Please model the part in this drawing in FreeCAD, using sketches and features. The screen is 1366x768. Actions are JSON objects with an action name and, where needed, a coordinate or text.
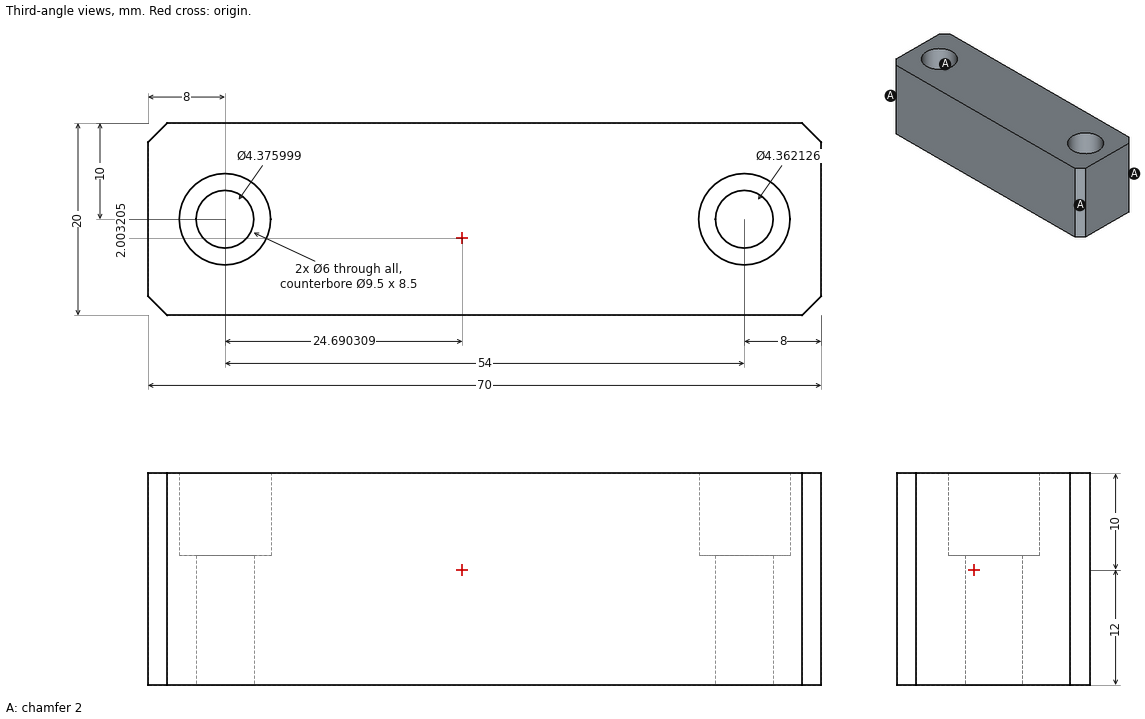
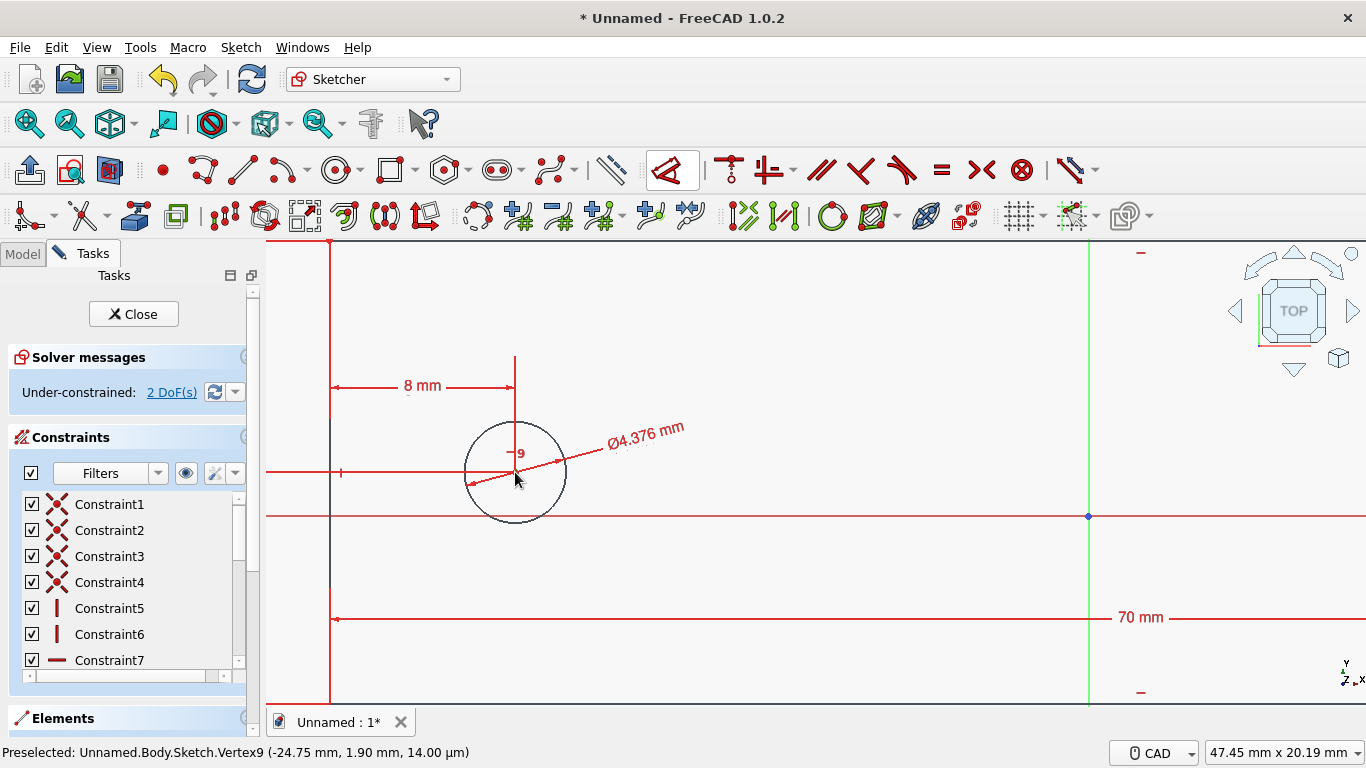
{"action": "key", "text": "i"}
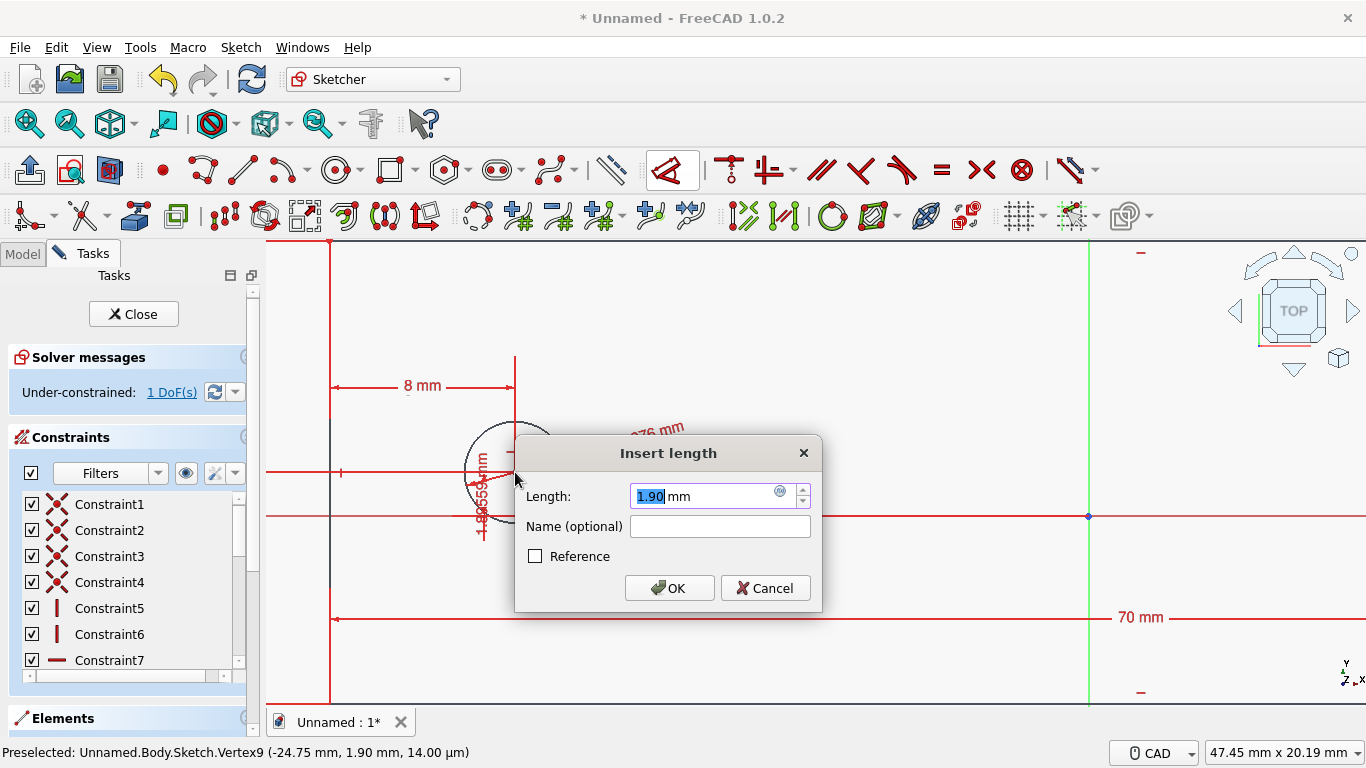
{"action": "type", "text": "2.003205"}
{"action": "key", "text": "Return"}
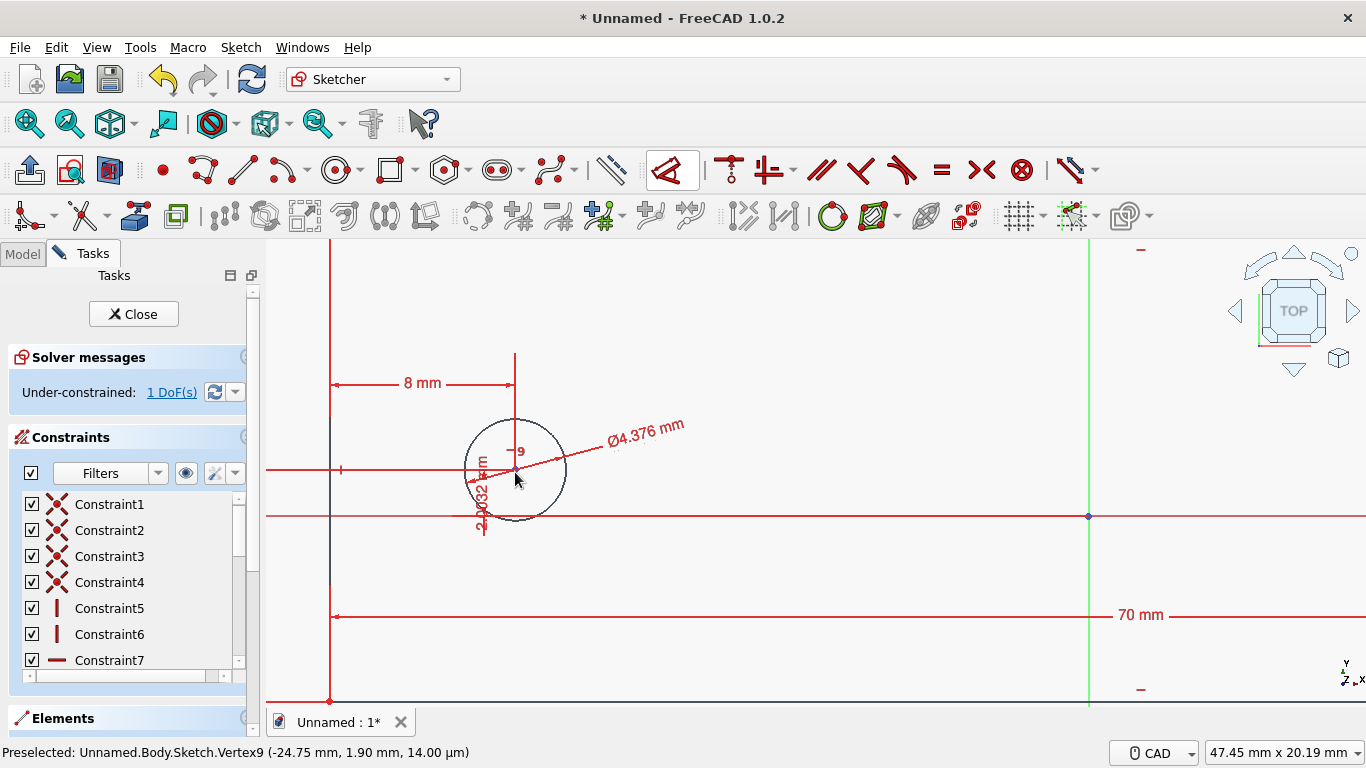
{"action": "left_click", "coordinate": [515, 470]}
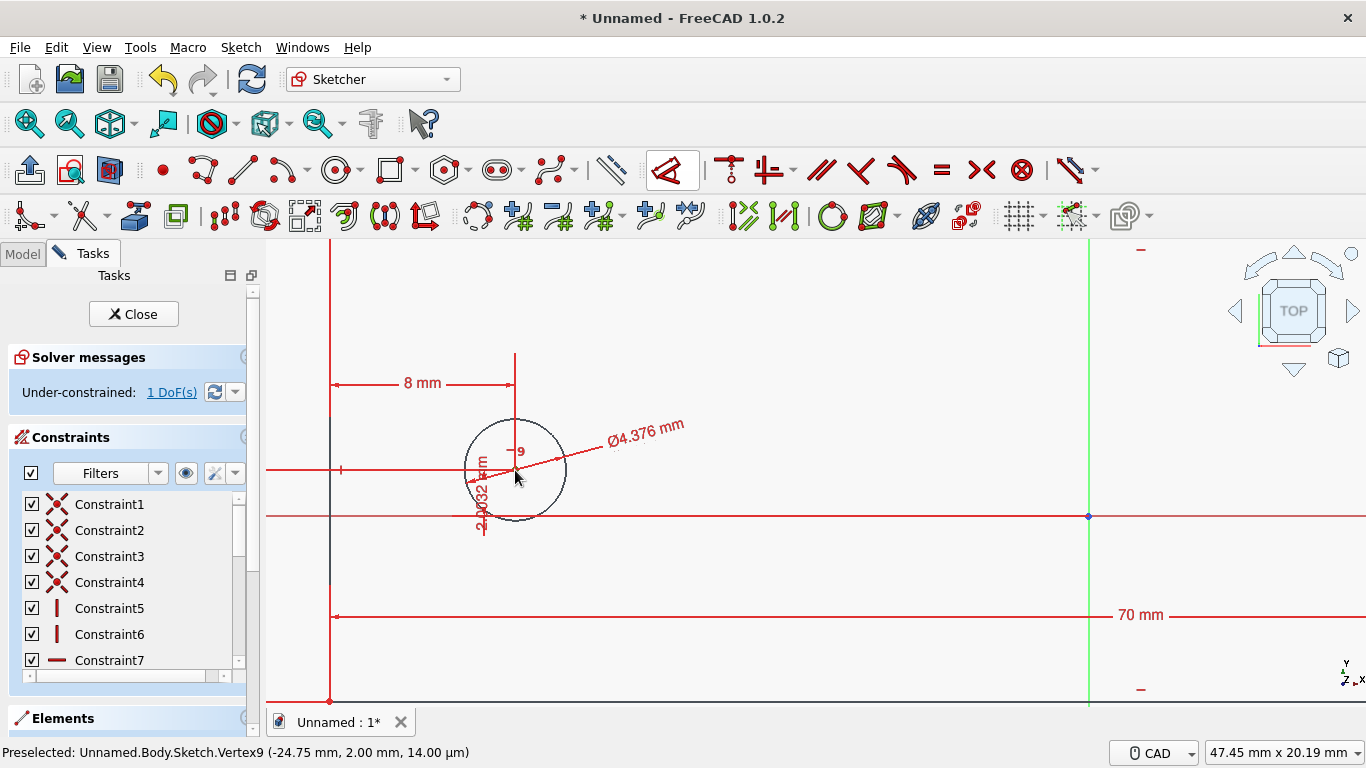
{"action": "key", "text": "l"}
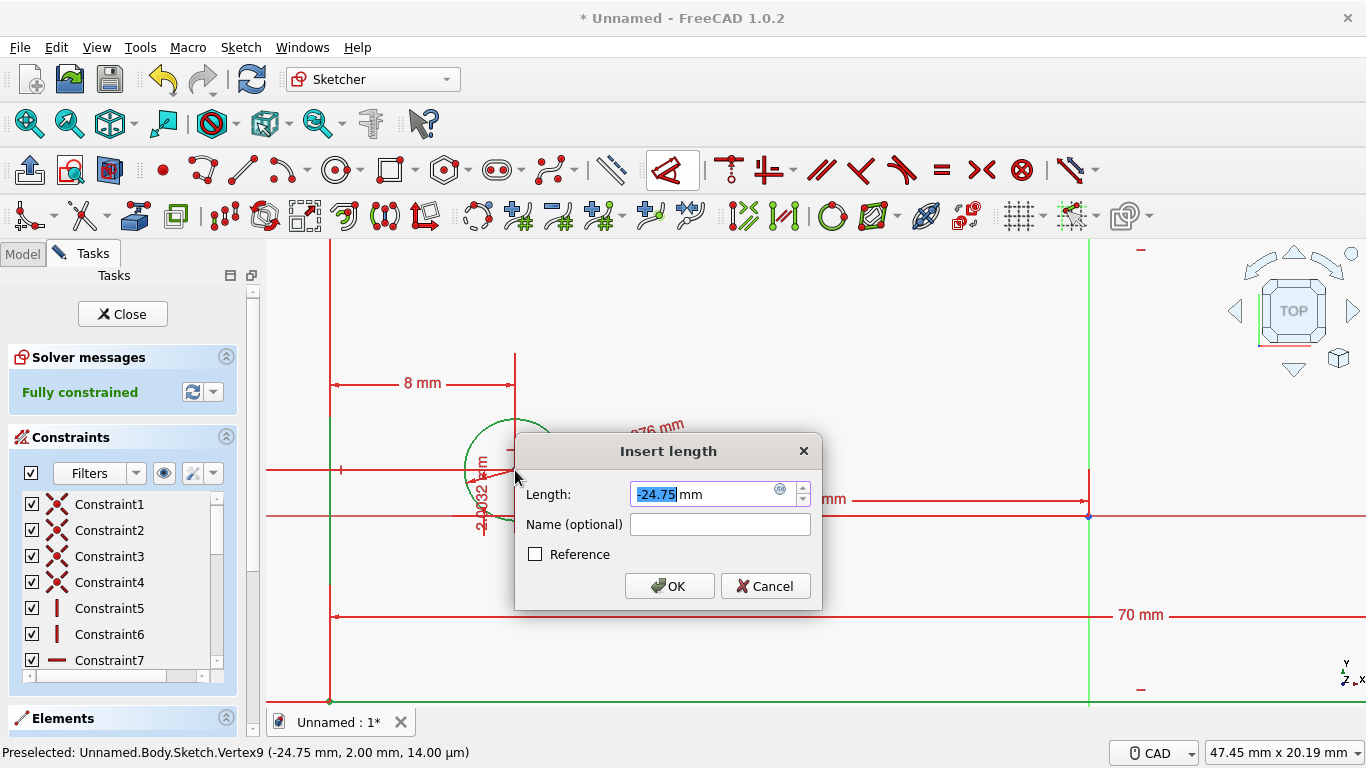
{"action": "type", "text": "-24.690309"}
{"action": "key", "text": "Return"}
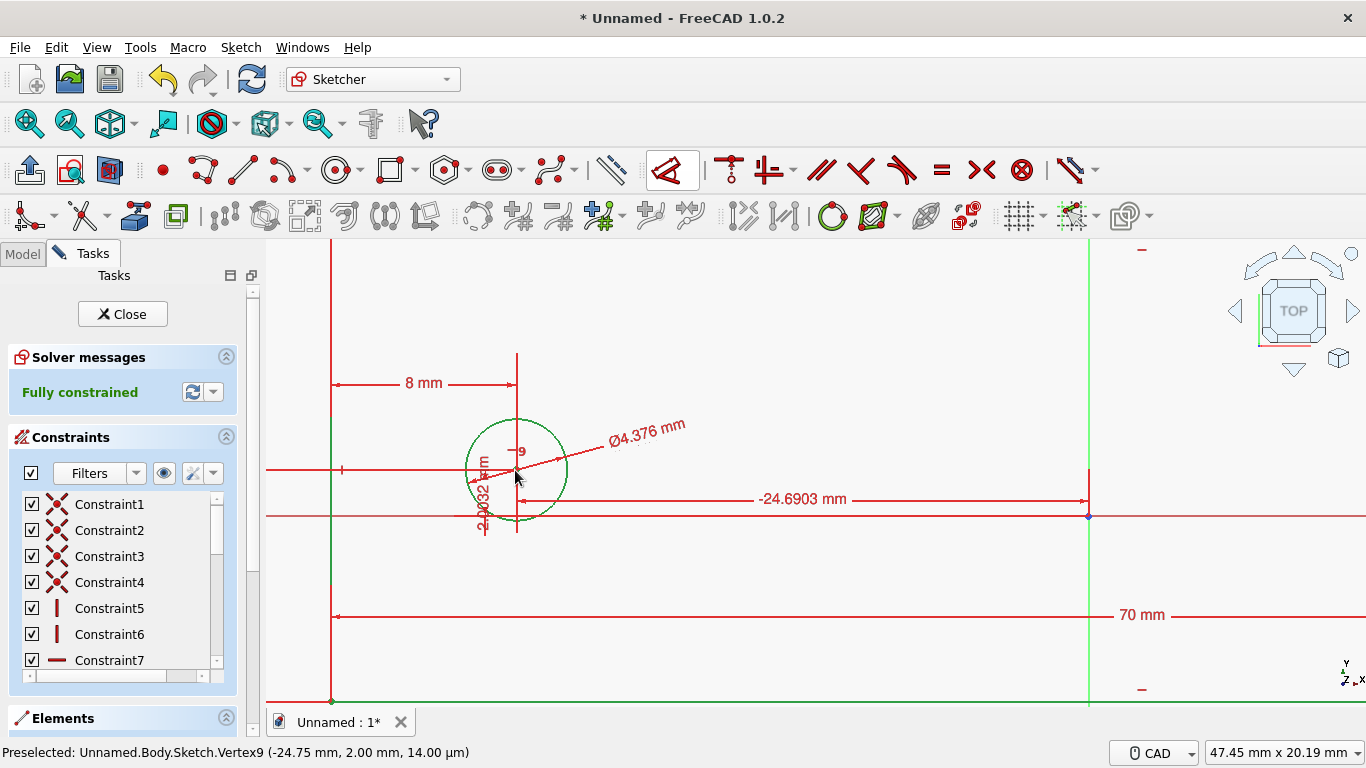
{"action": "left_click", "coordinate": [123, 314]}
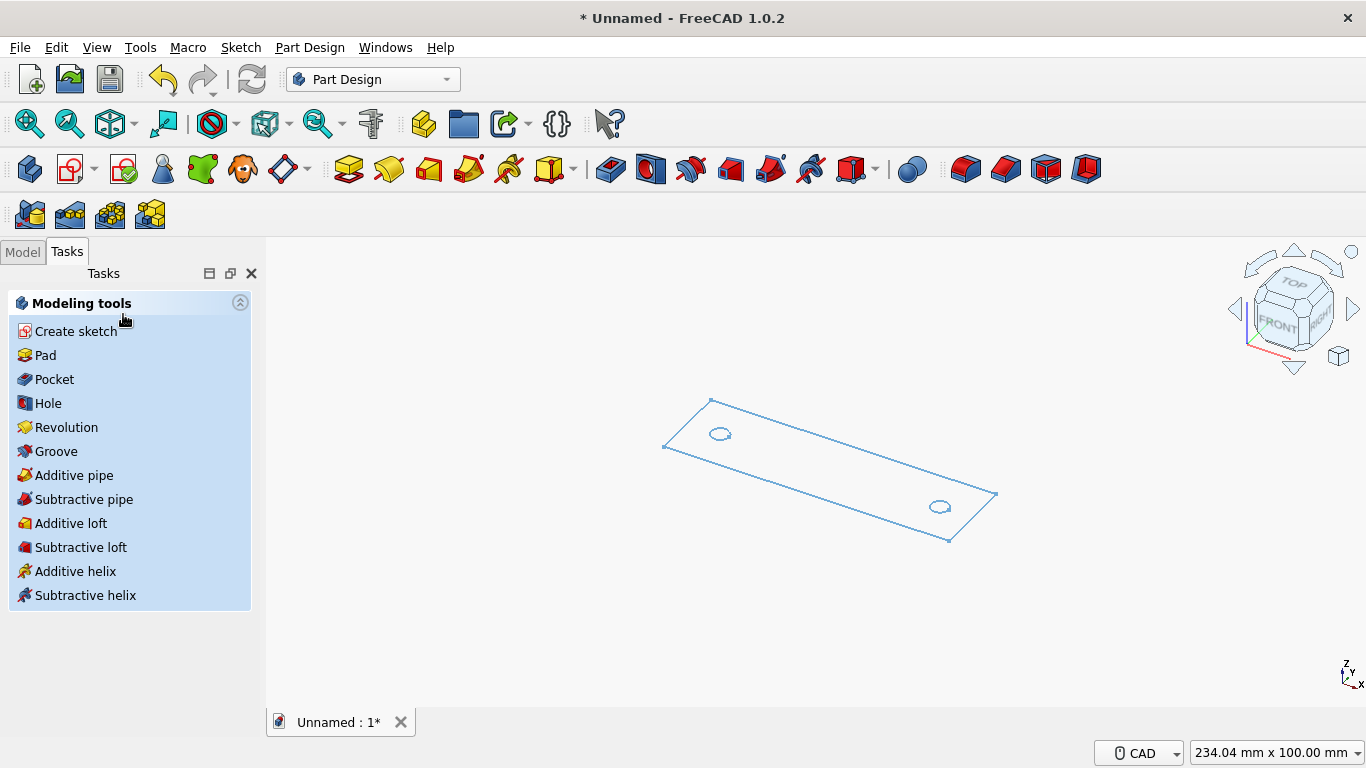
{"action": "left_click", "coordinate": [350, 170]}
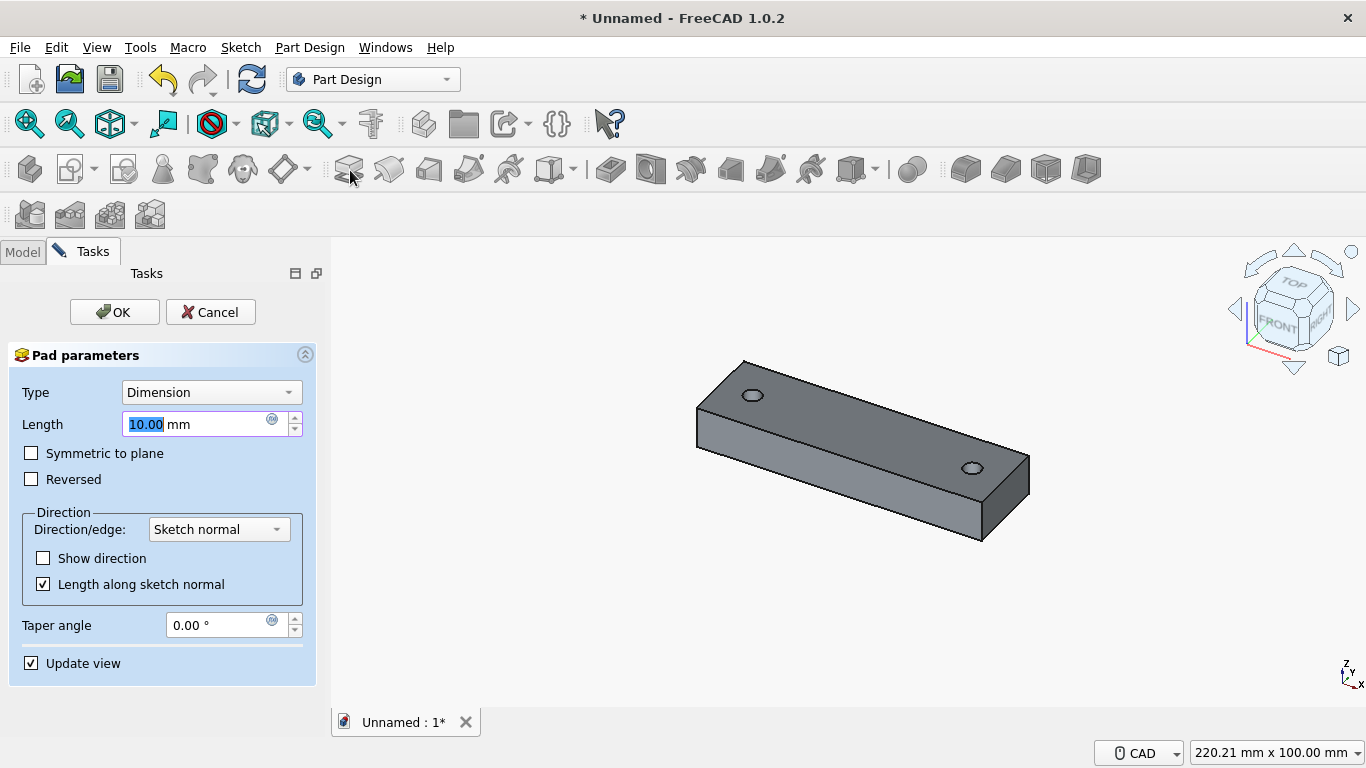
{"action": "left_click", "coordinate": [212, 392]}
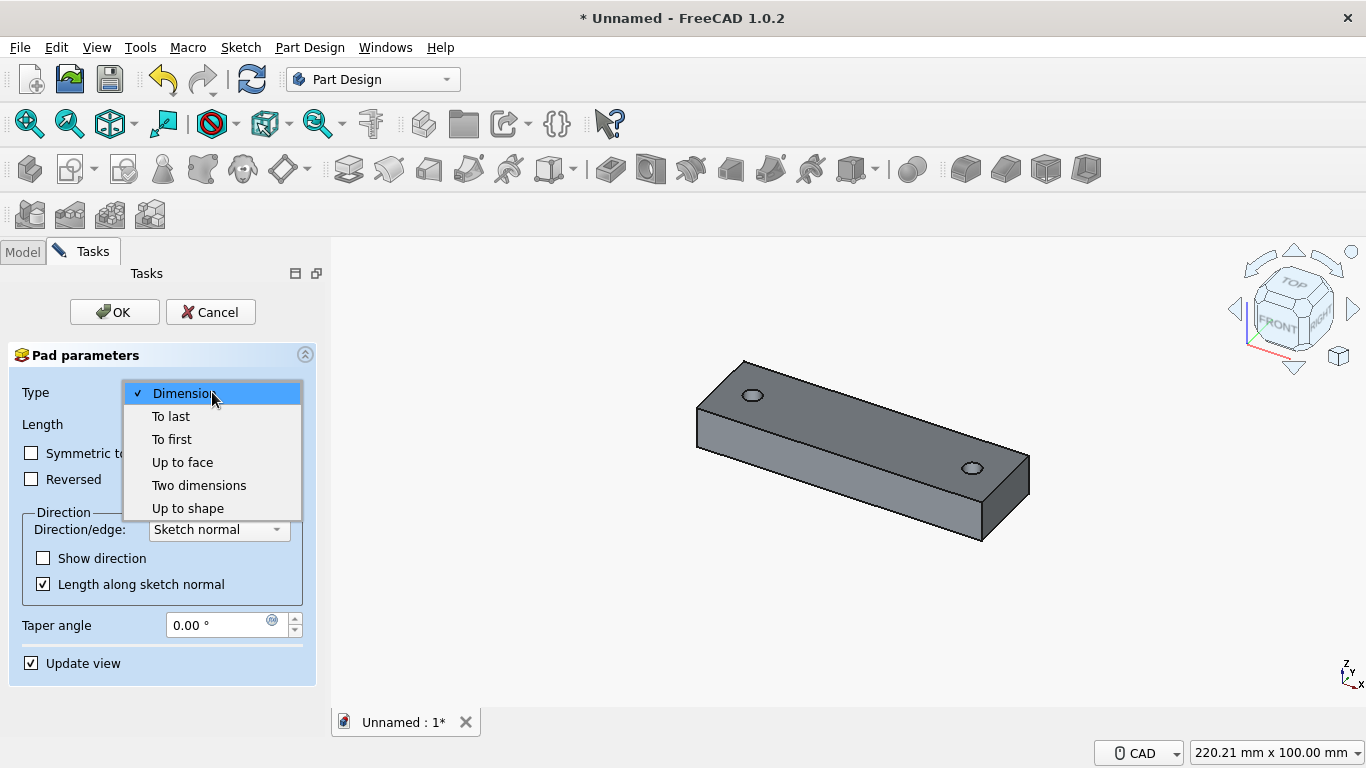
{"action": "left_click", "coordinate": [212, 486]}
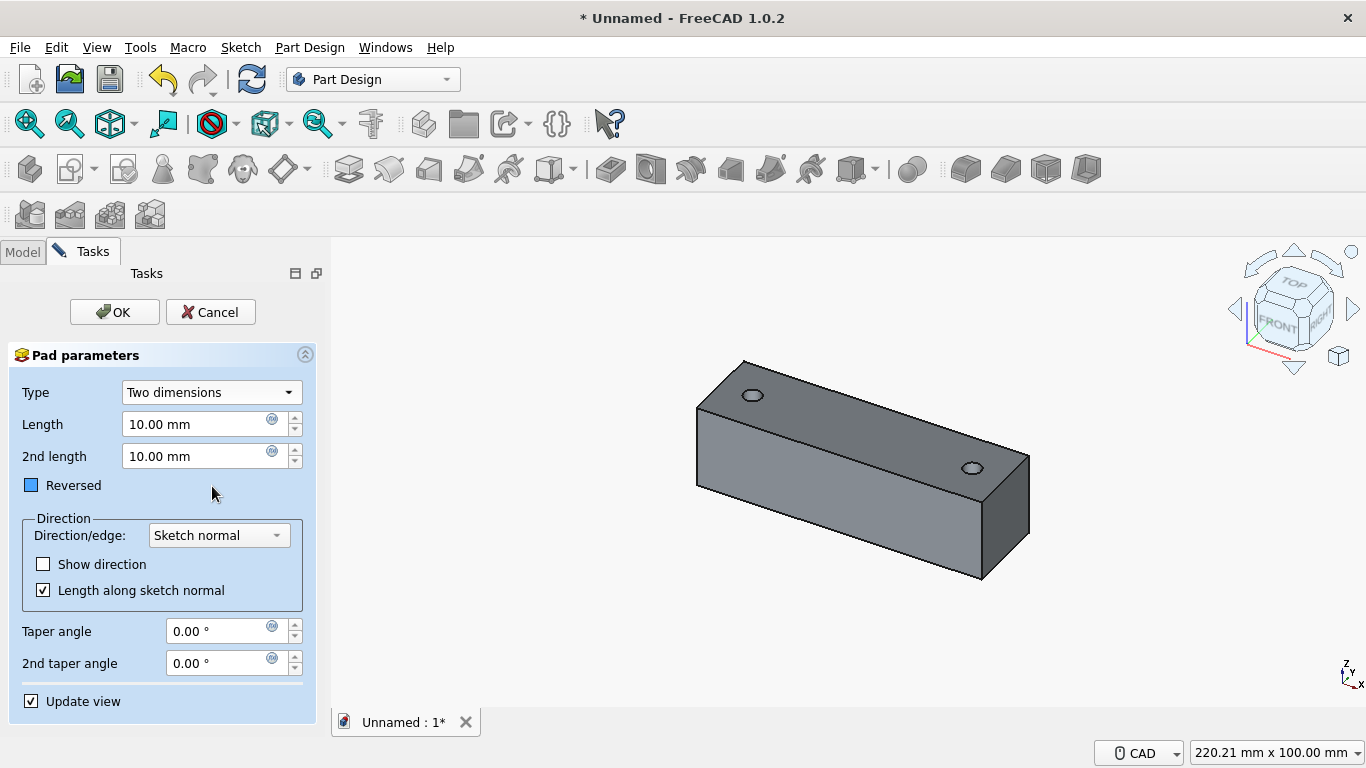
{"action": "triple_click", "coordinate": [204, 424]}